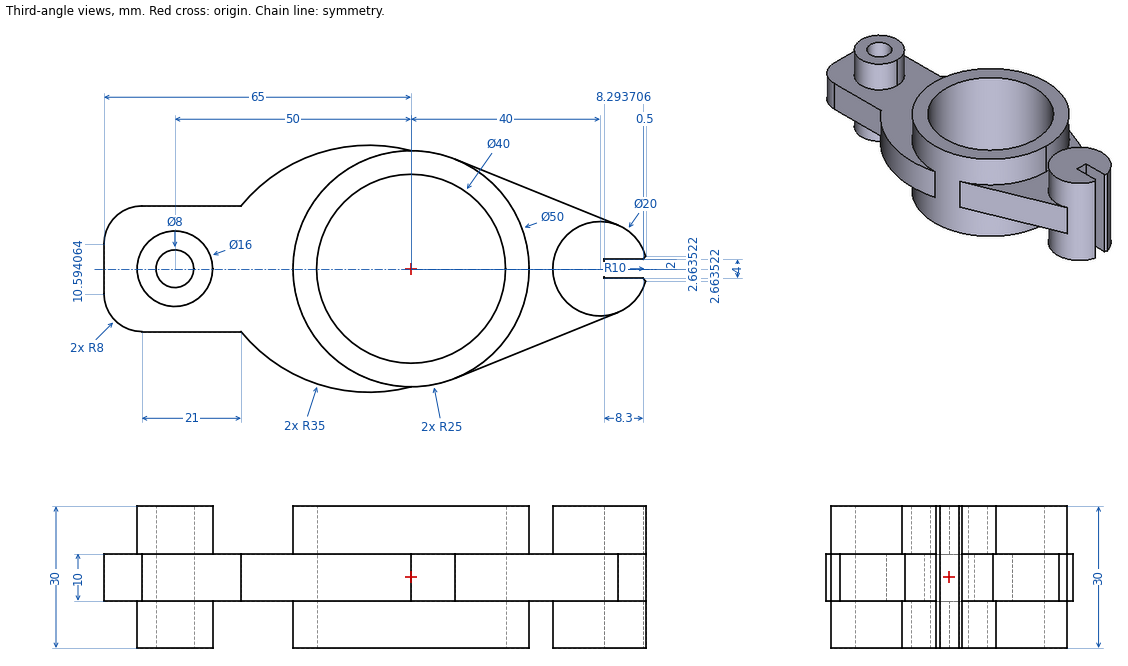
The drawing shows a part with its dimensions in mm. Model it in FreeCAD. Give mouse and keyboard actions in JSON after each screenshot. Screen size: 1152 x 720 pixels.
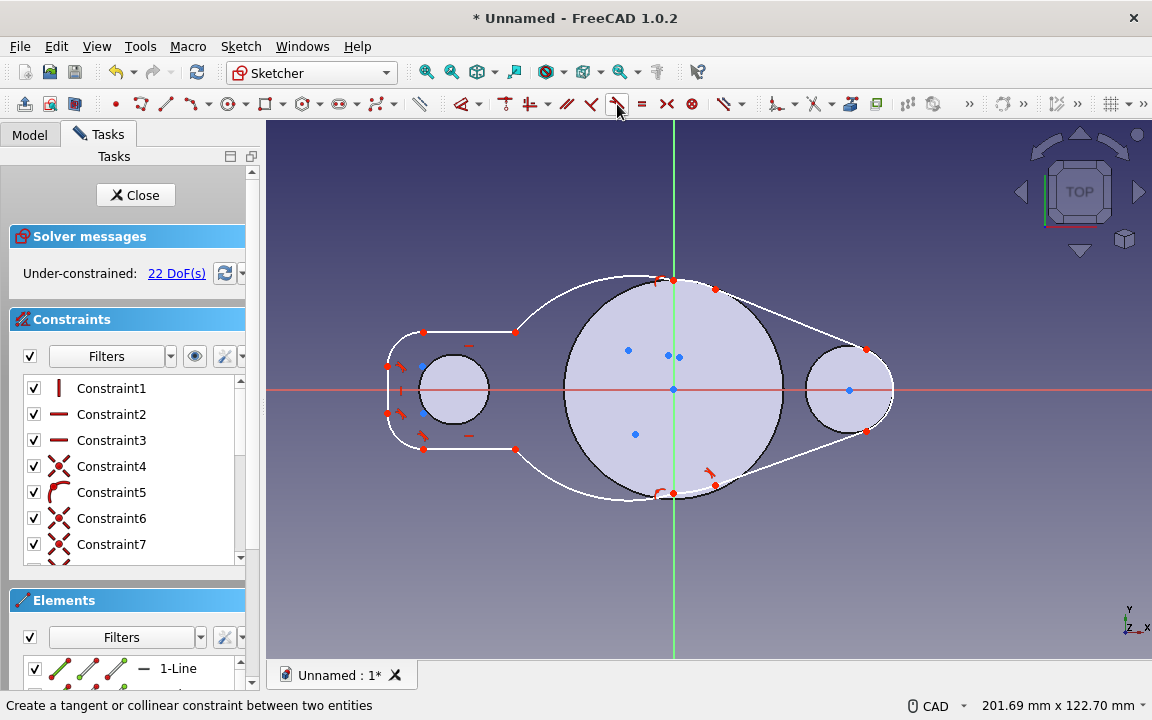
{"action": "left_click", "coordinate": [760, 469]}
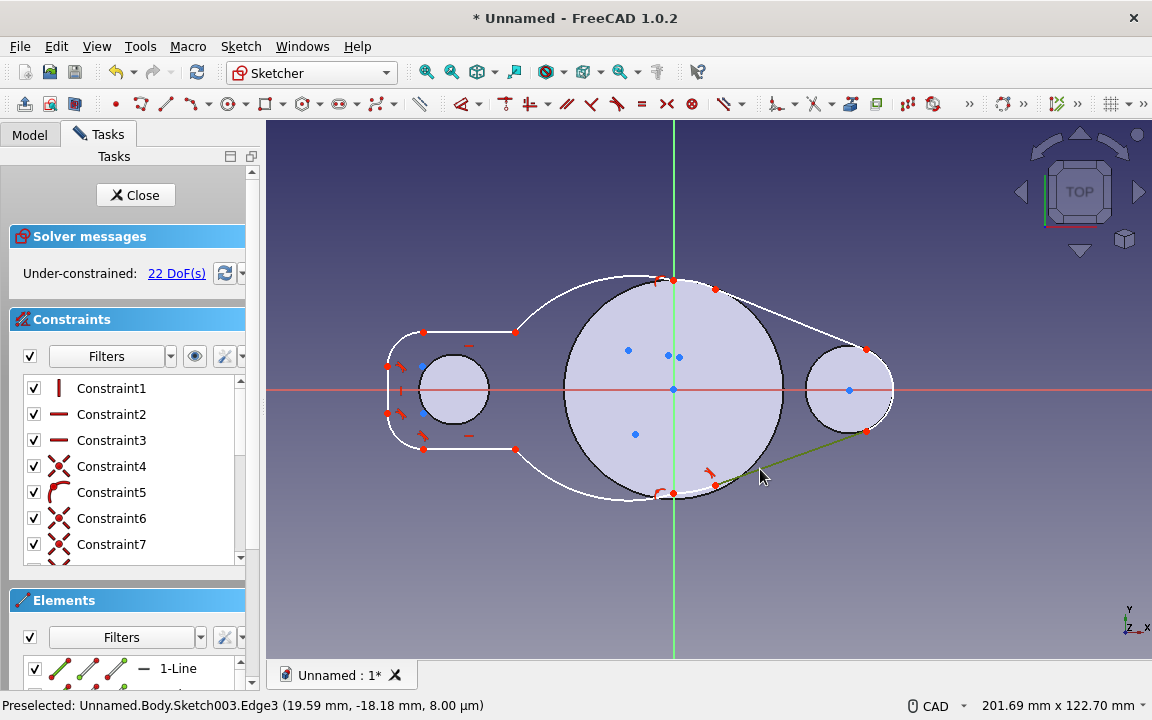
{"action": "left_click", "coordinate": [889, 410]}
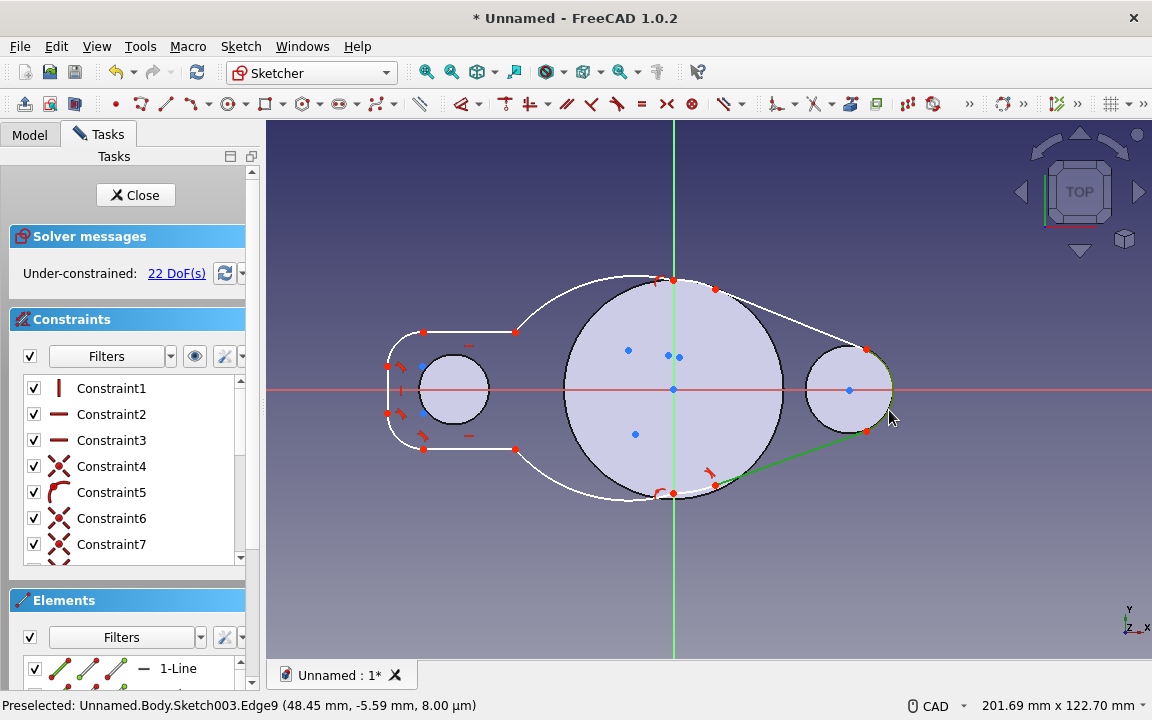
{"action": "left_click", "coordinate": [617, 104]}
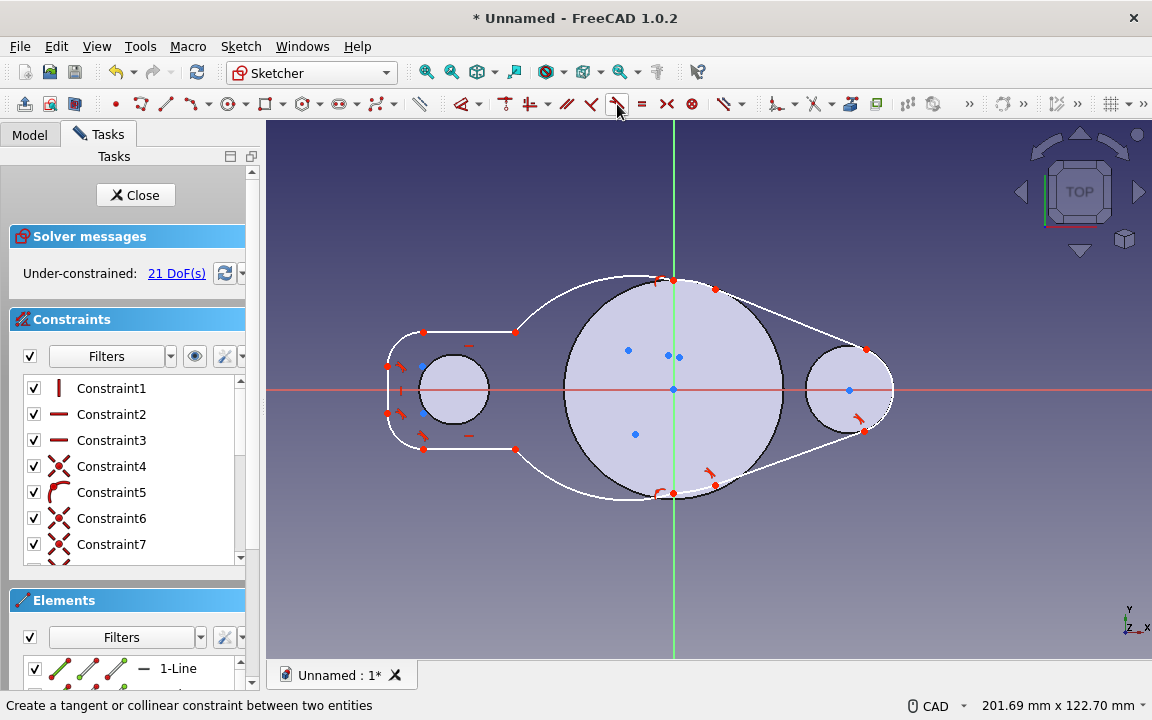
{"action": "left_click", "coordinate": [821, 332]}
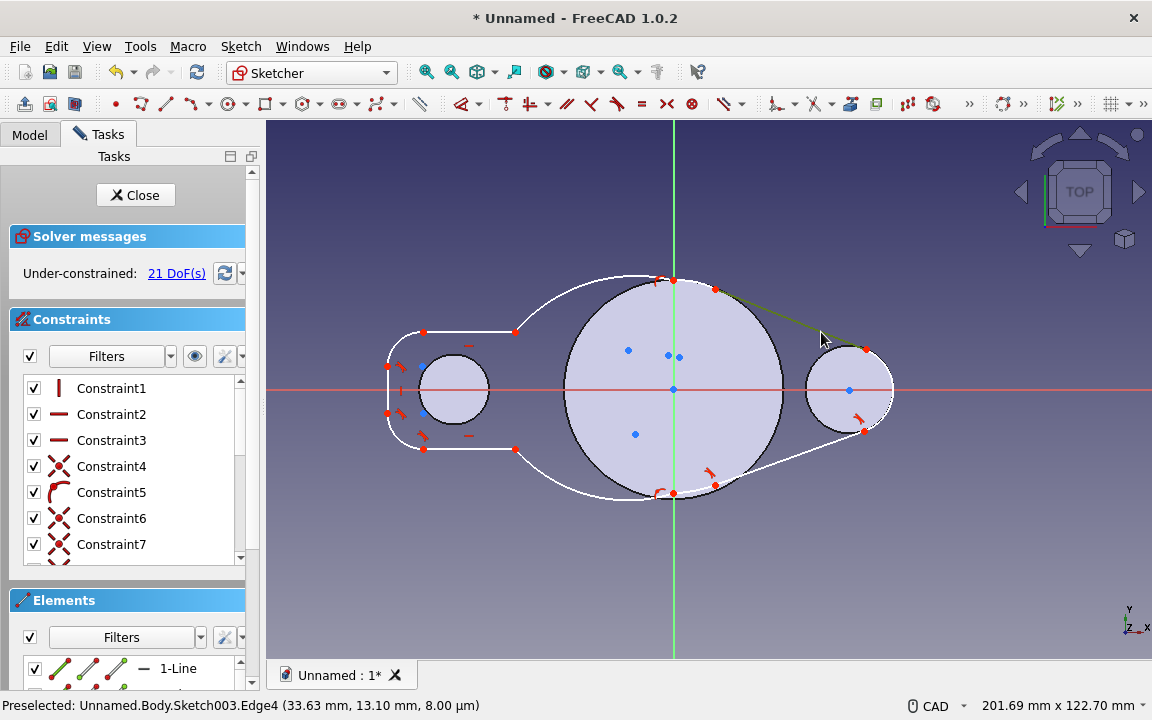
{"action": "left_click", "coordinate": [888, 411]}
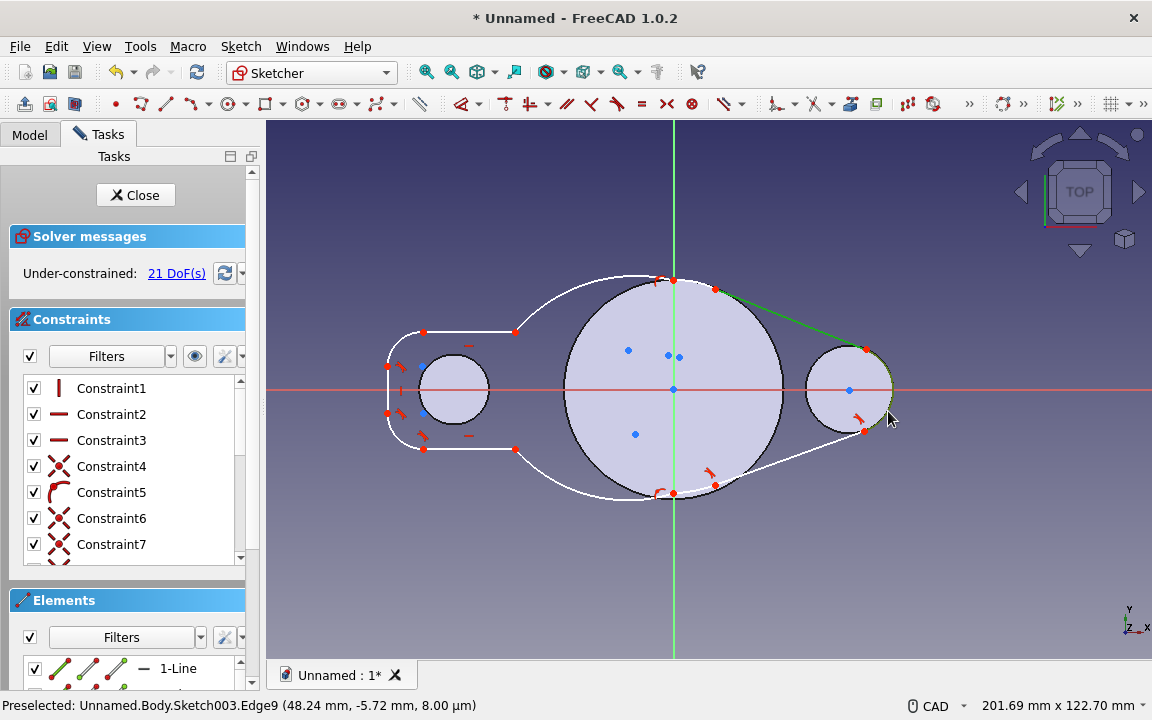
{"action": "left_click", "coordinate": [617, 104]}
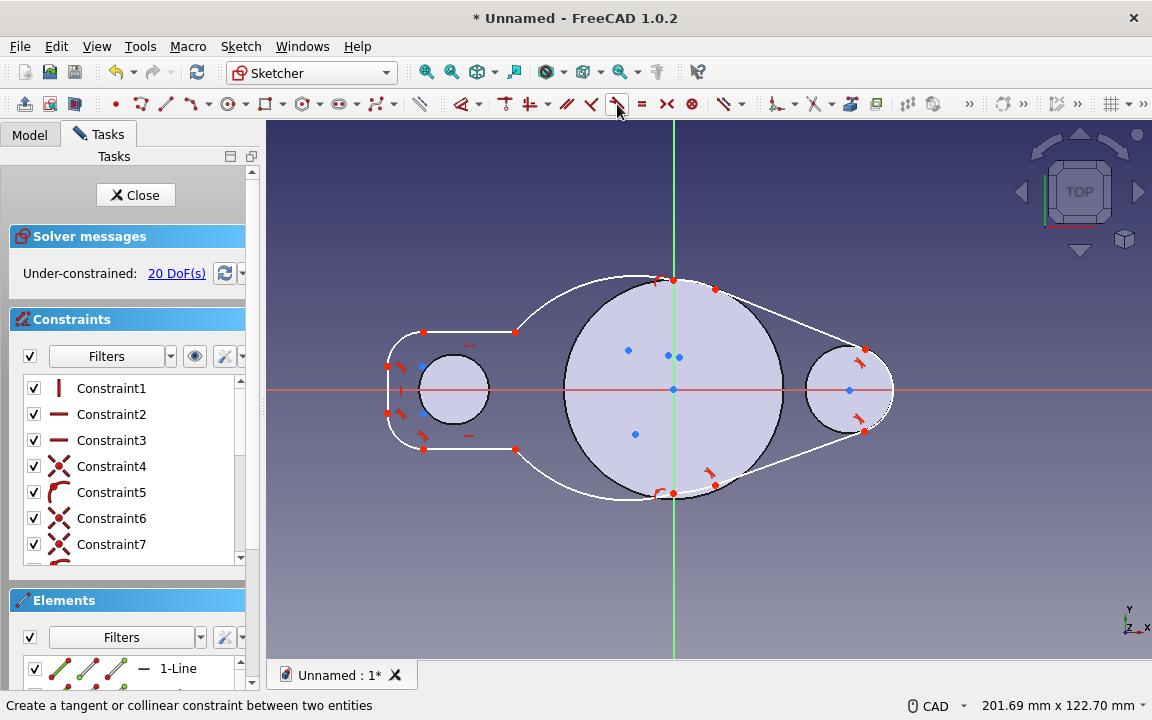
{"action": "left_click", "coordinate": [821, 332]}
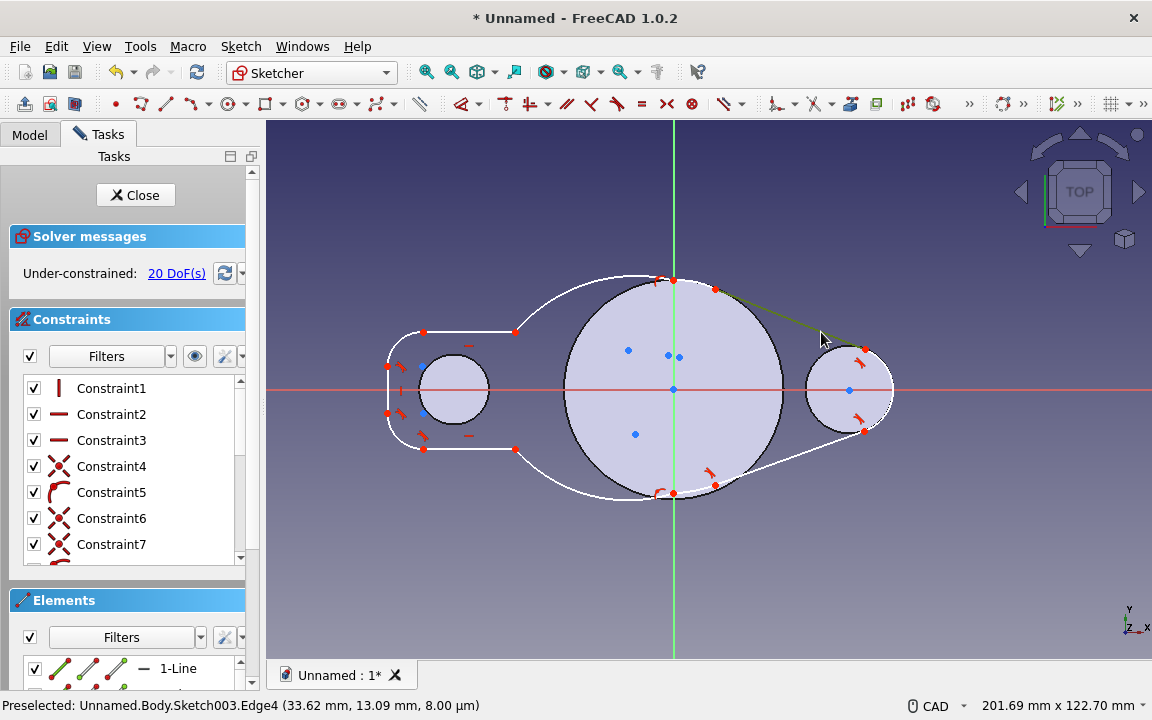
{"action": "left_click", "coordinate": [703, 284]}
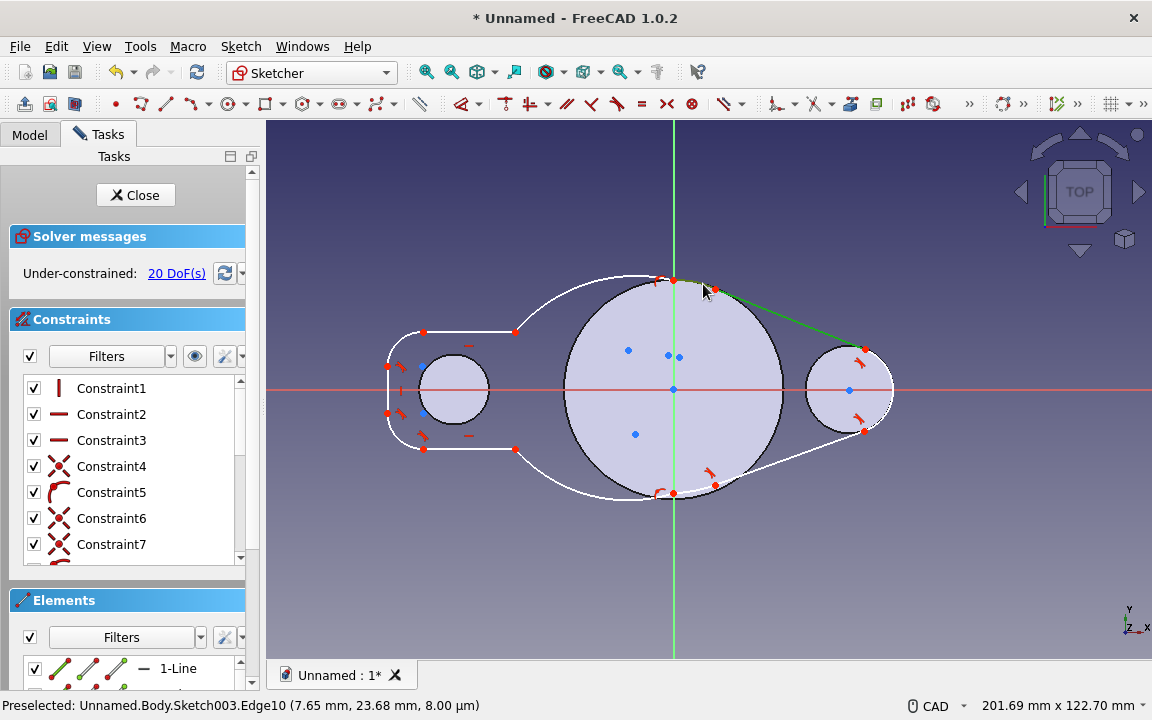
{"action": "left_click", "coordinate": [617, 104]}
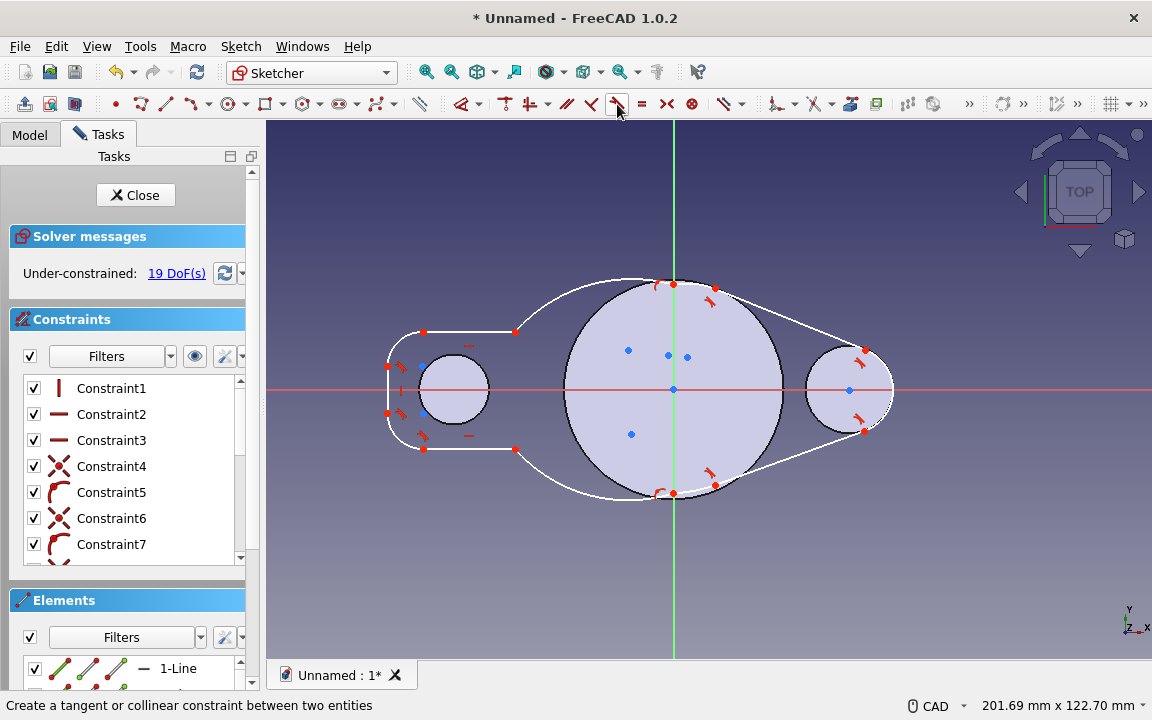
{"action": "left_click", "coordinate": [488, 332]}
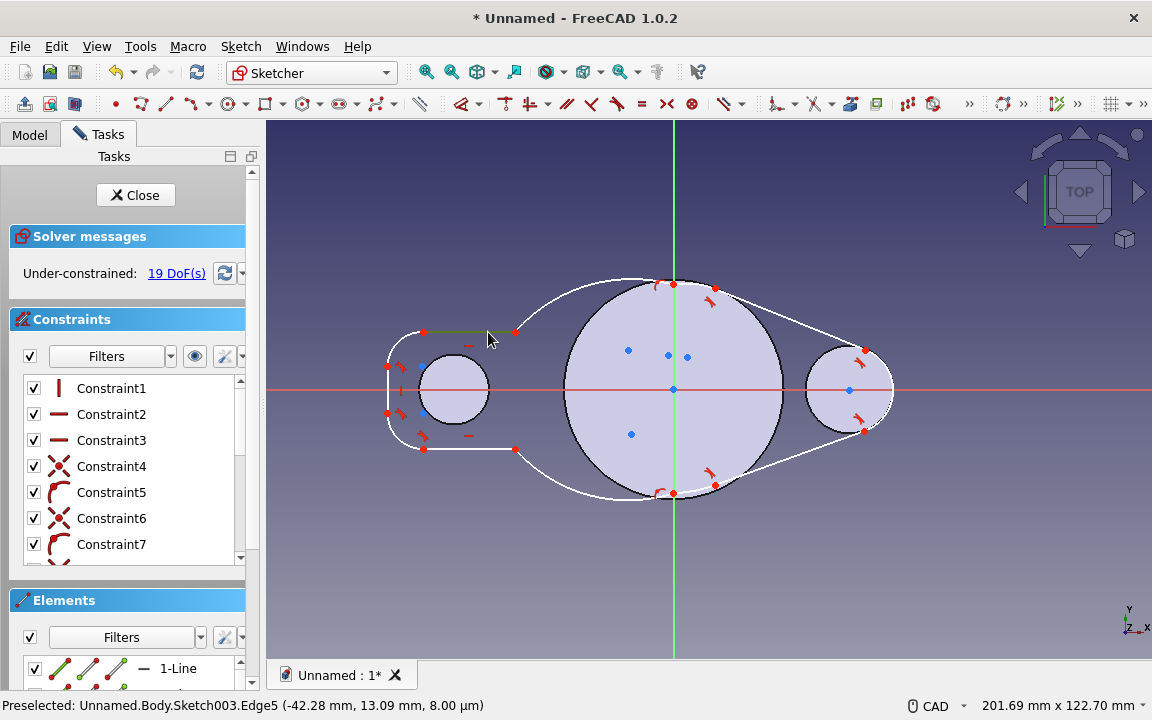
{"action": "left_click", "coordinate": [407, 336]}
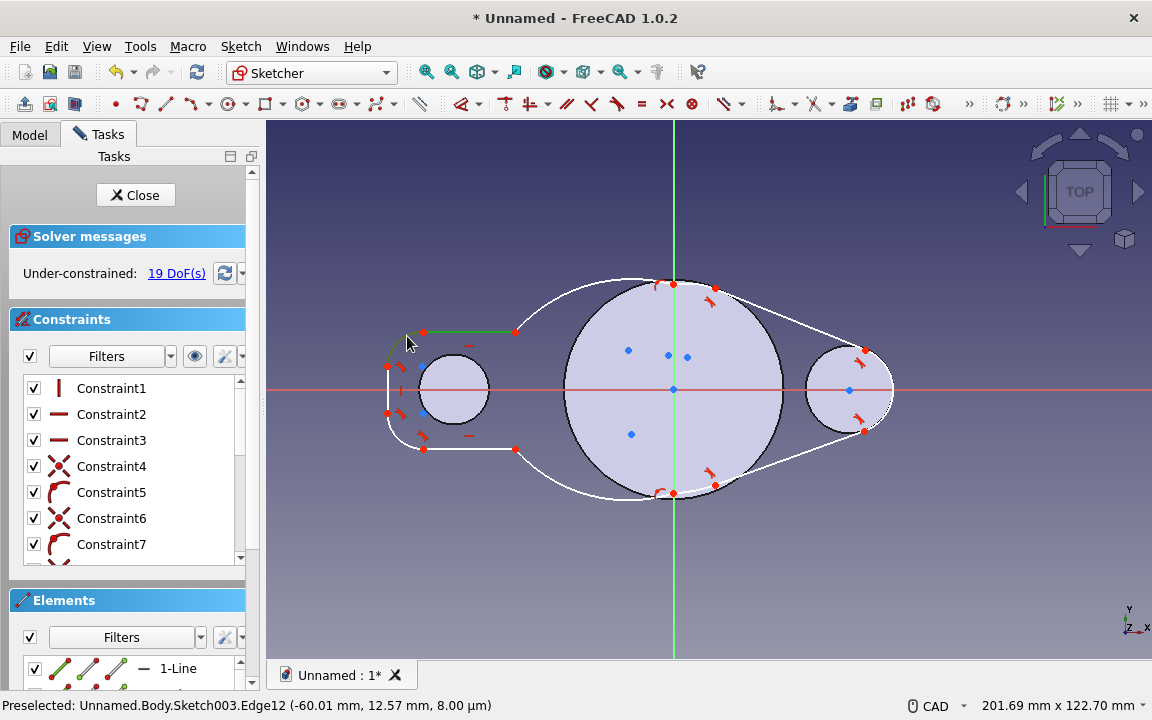
{"action": "left_click", "coordinate": [617, 104]}